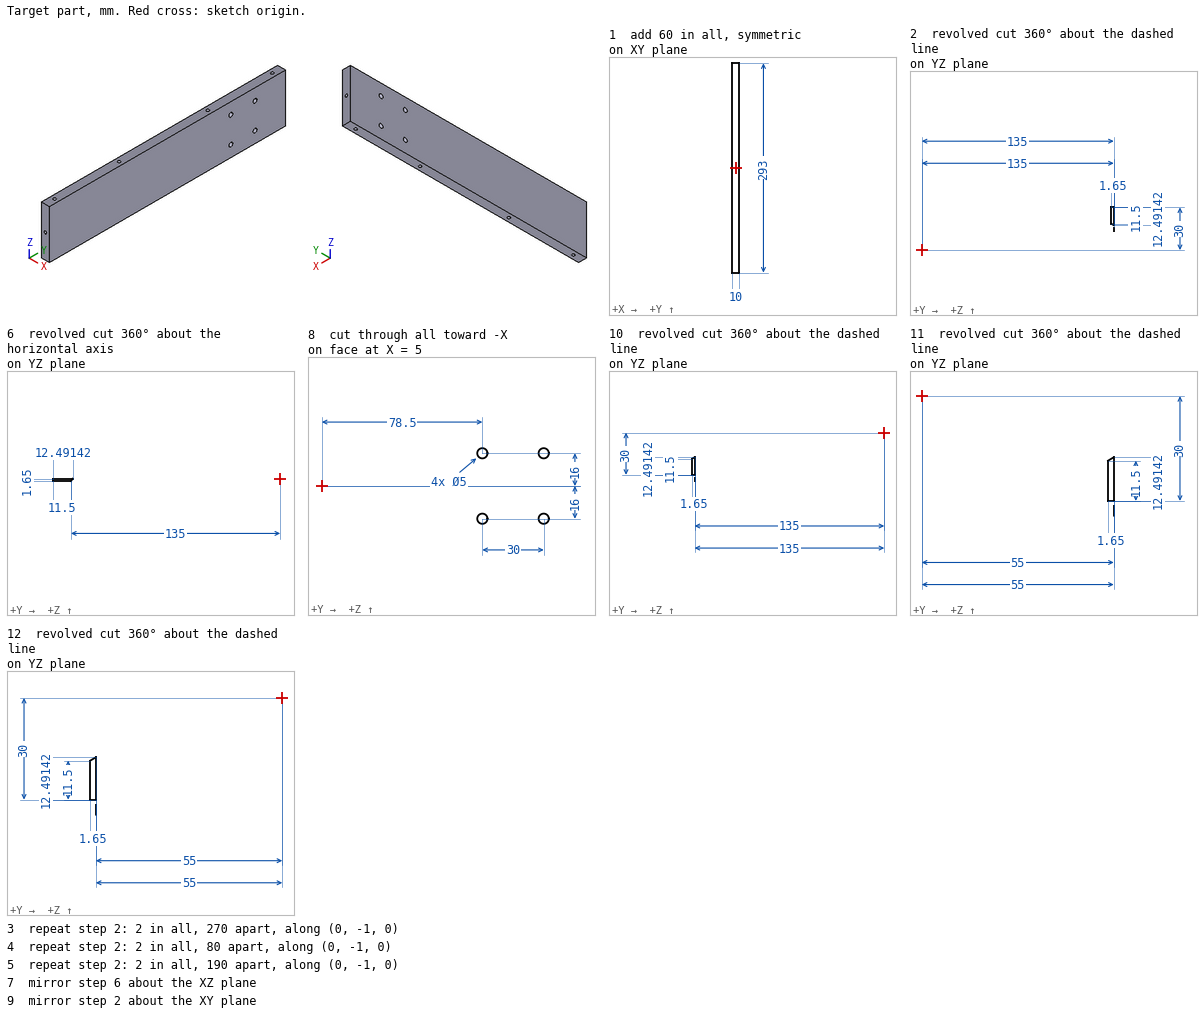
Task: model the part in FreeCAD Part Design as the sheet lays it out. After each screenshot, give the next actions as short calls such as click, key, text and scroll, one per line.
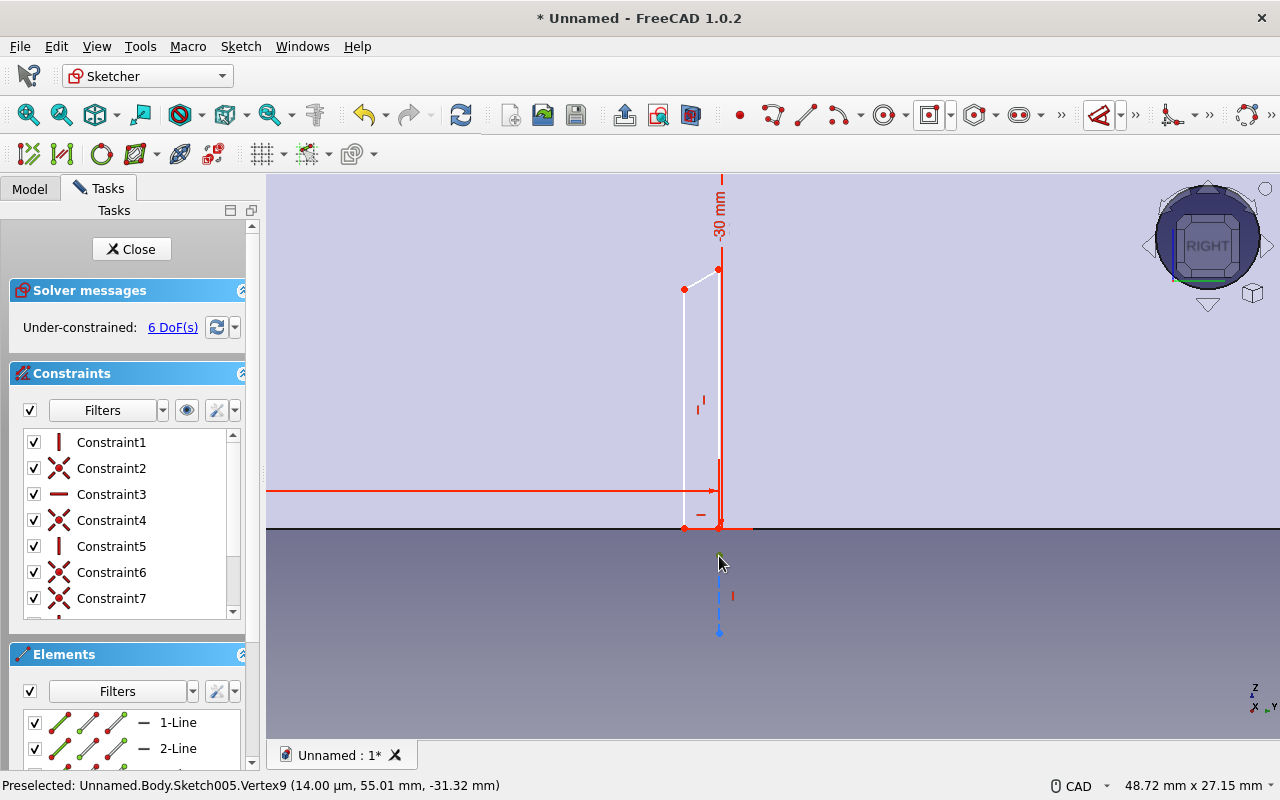
click(1120, 116)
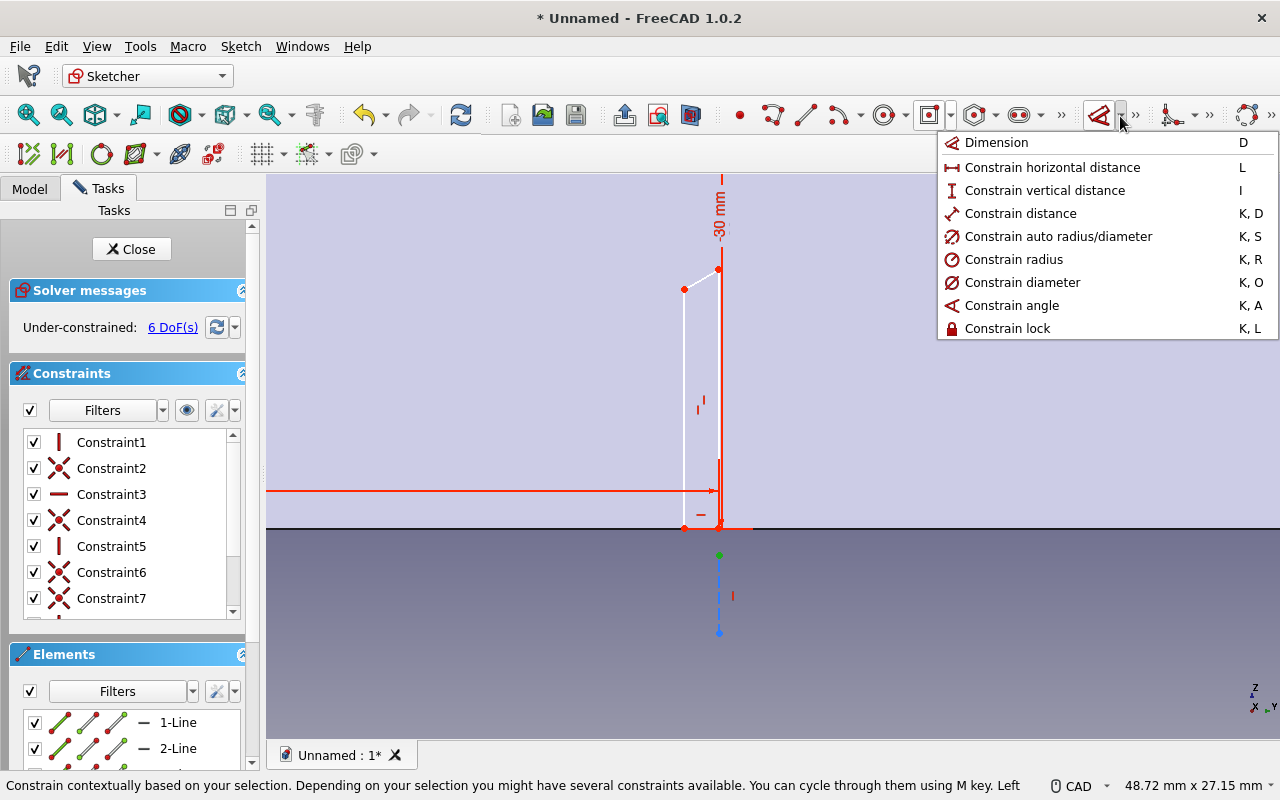
click(1108, 168)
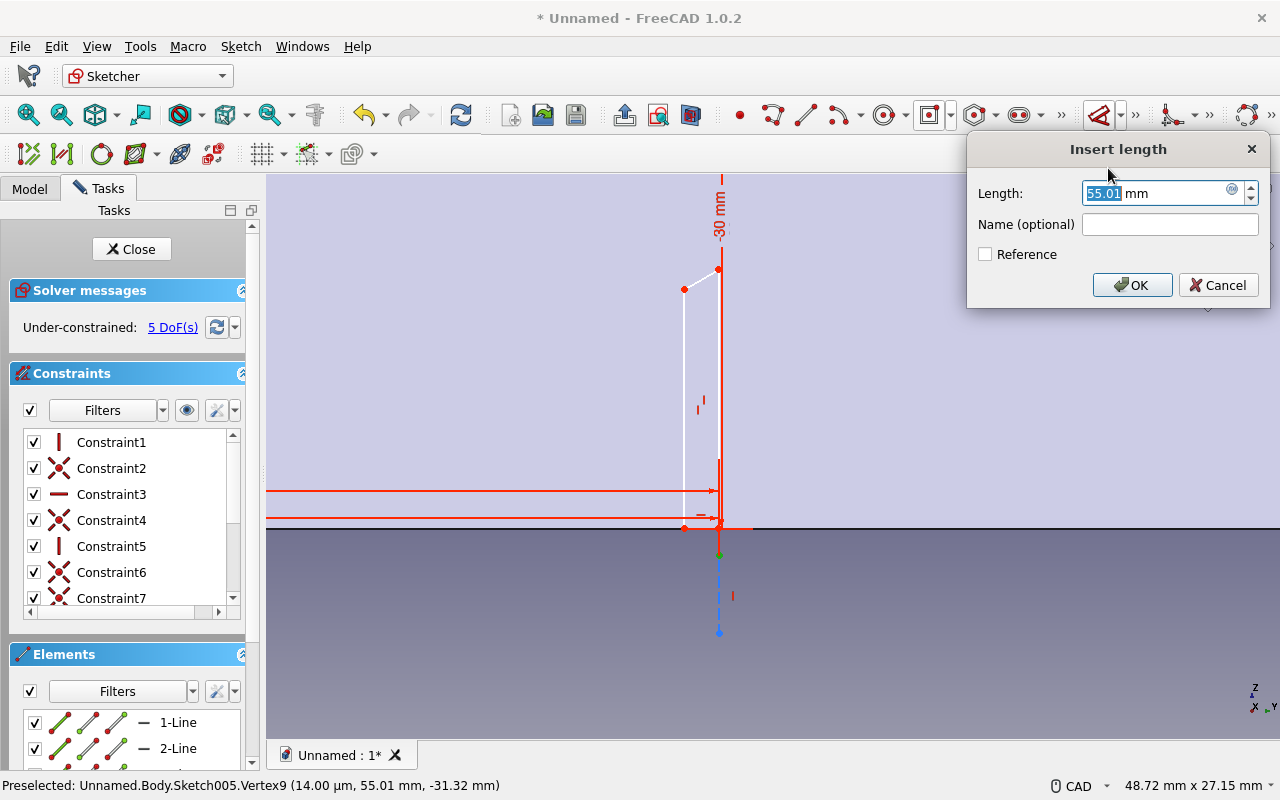
text(55)
key(Return)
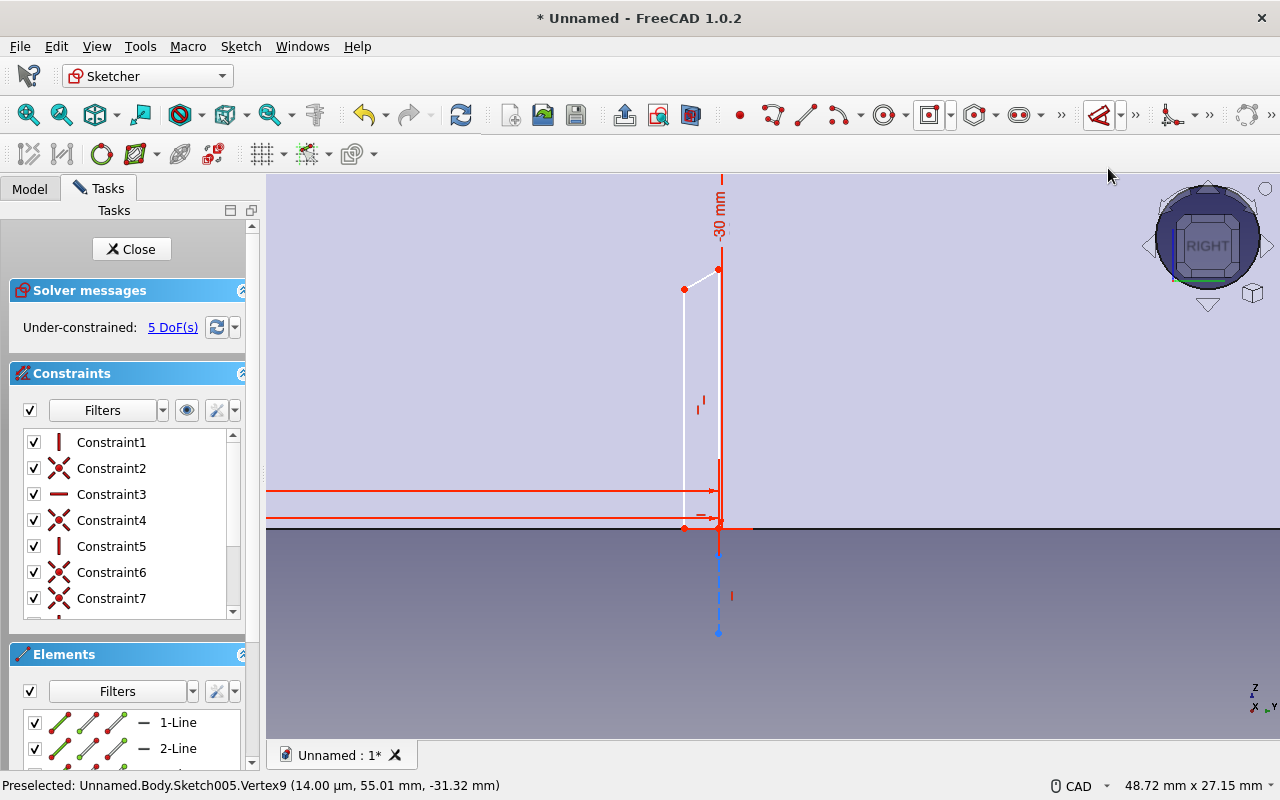
click(684, 362)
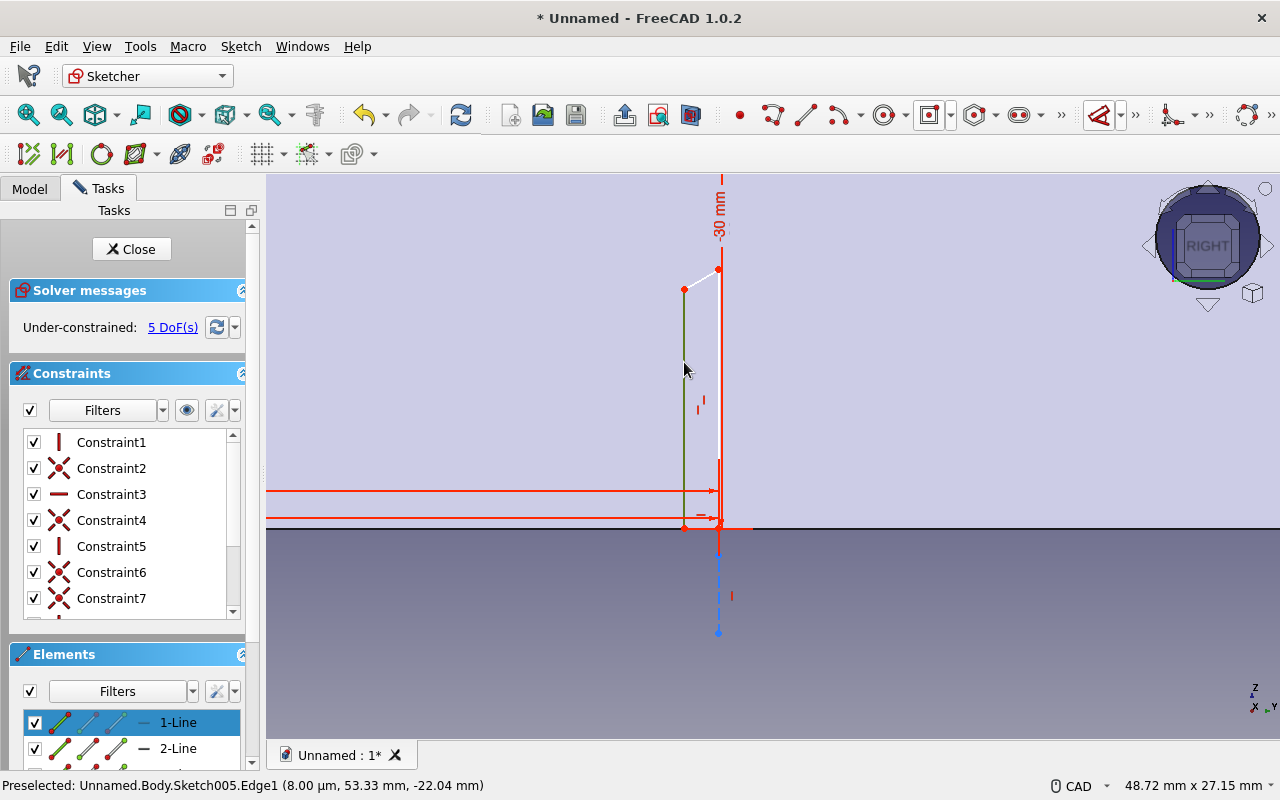
click(1120, 116)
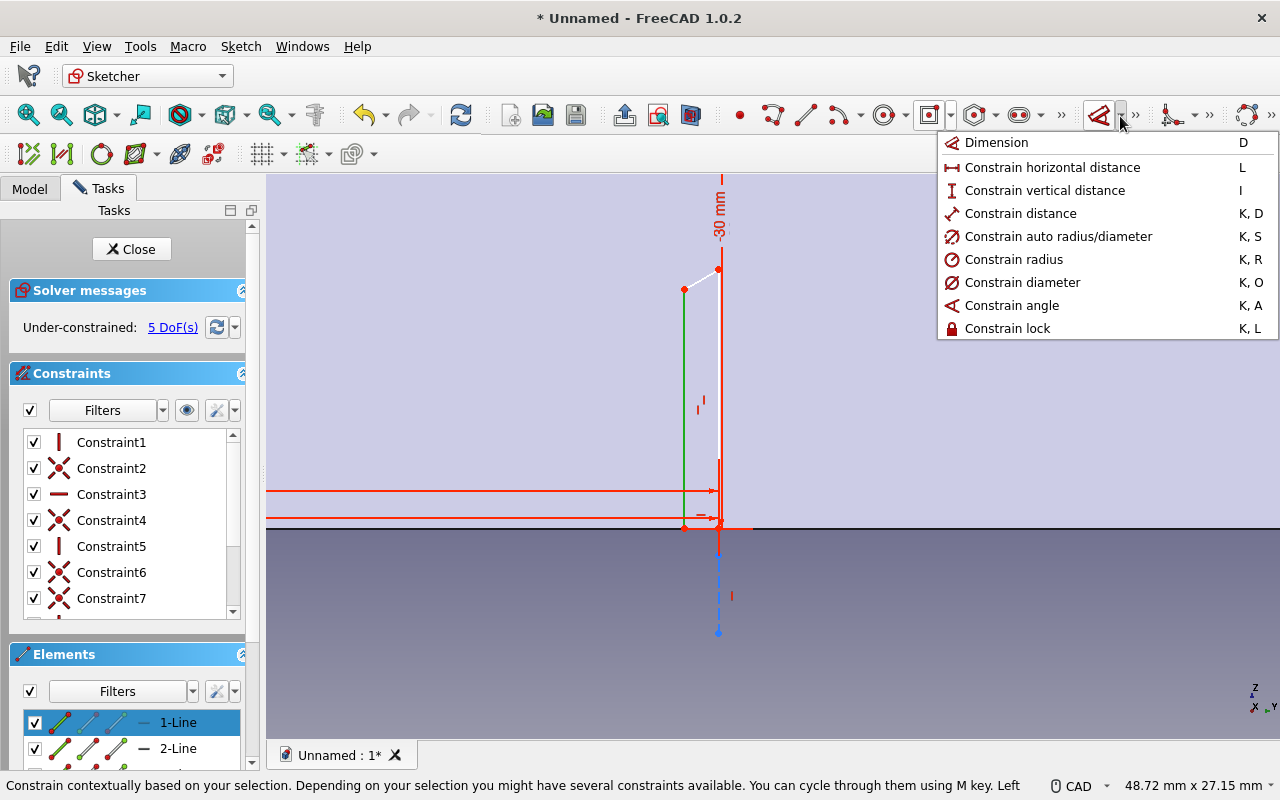
click(1108, 190)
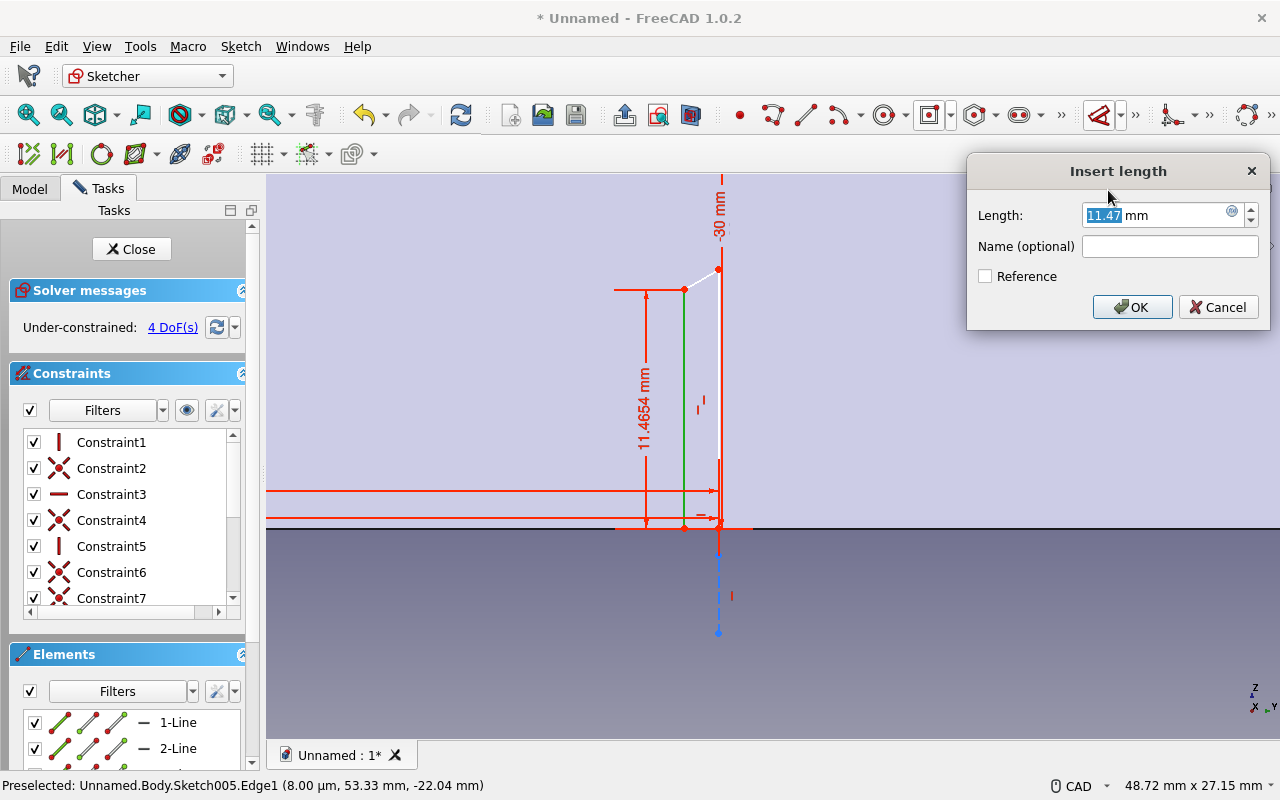
text(11.5)
key(Return)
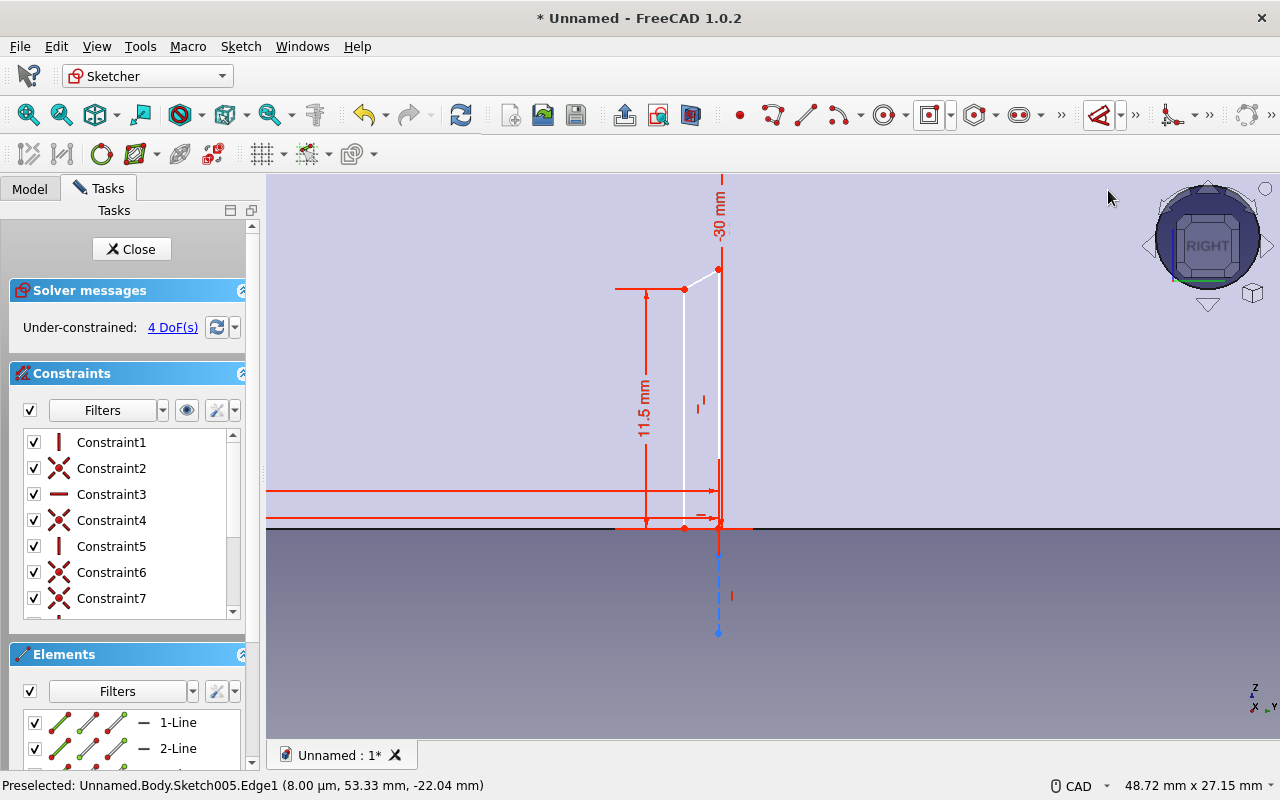
scroll(694, 529, up, 2)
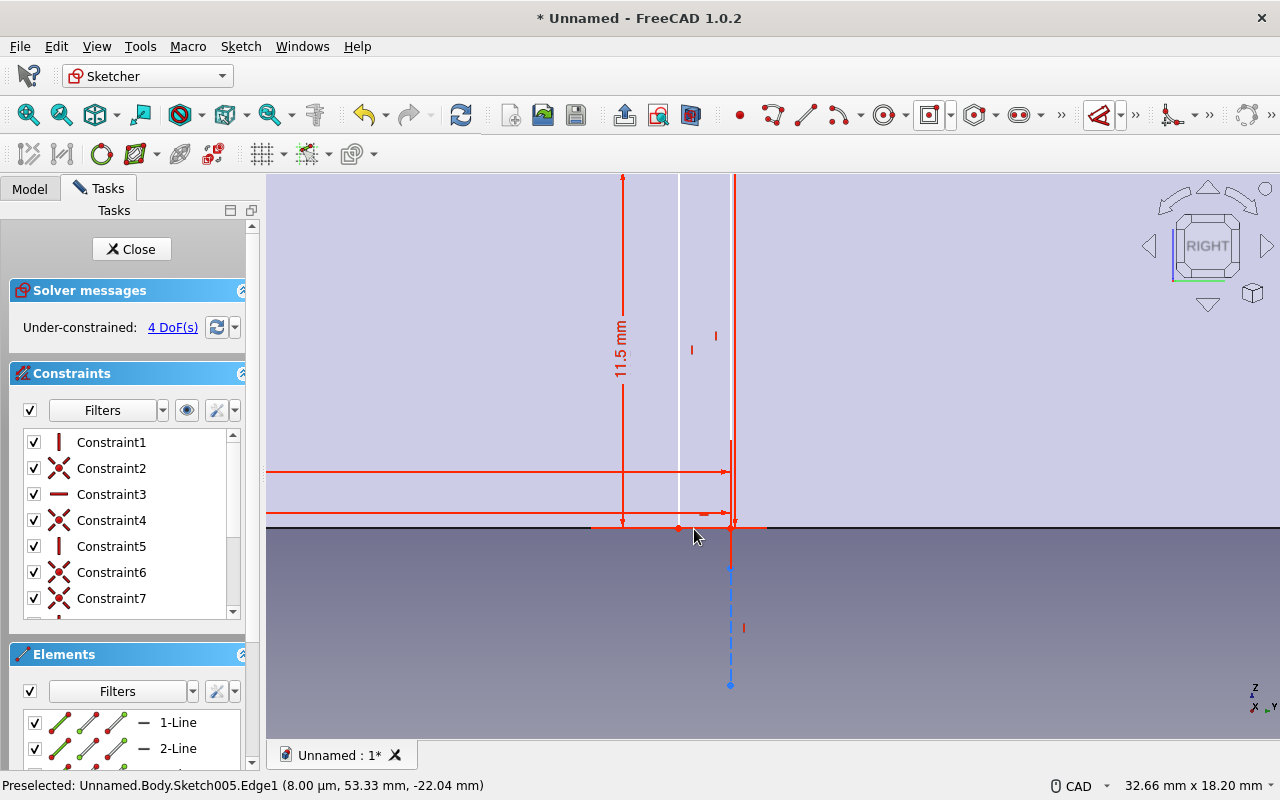
click(694, 528)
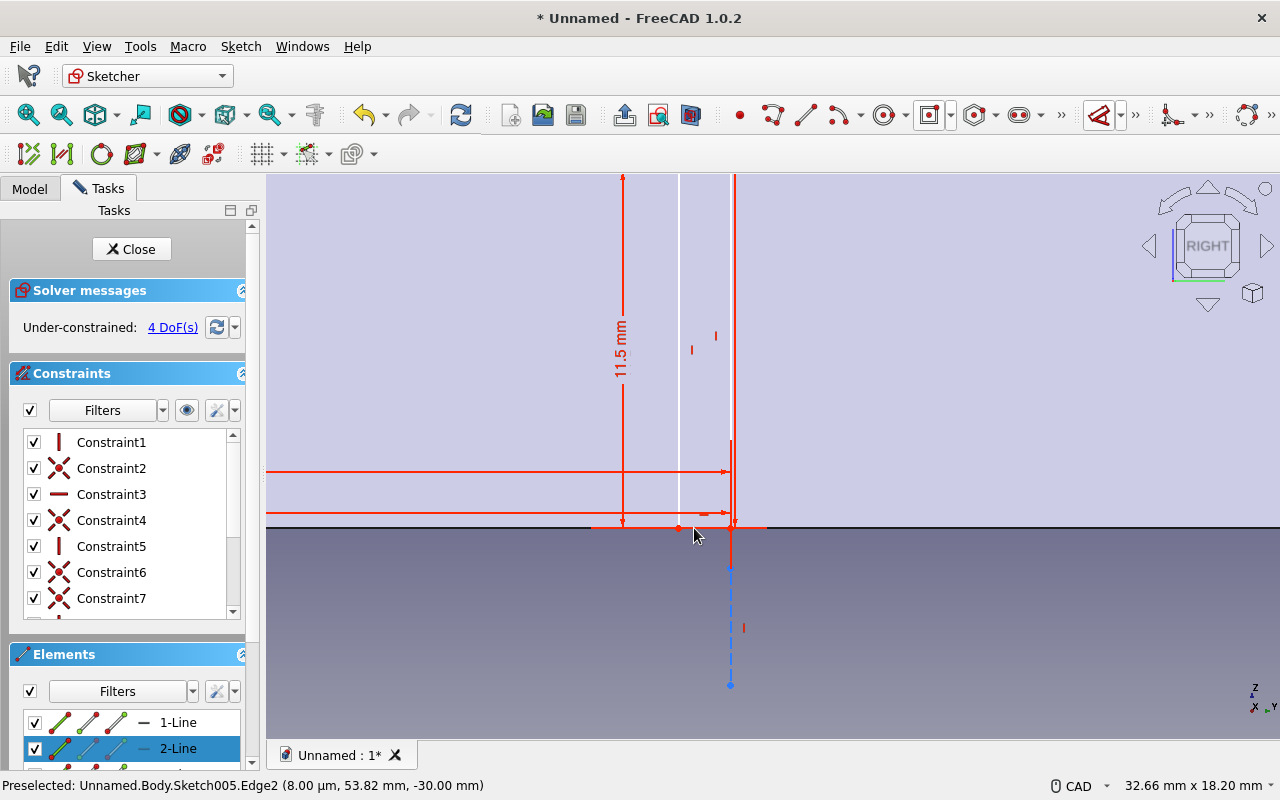
key(l)